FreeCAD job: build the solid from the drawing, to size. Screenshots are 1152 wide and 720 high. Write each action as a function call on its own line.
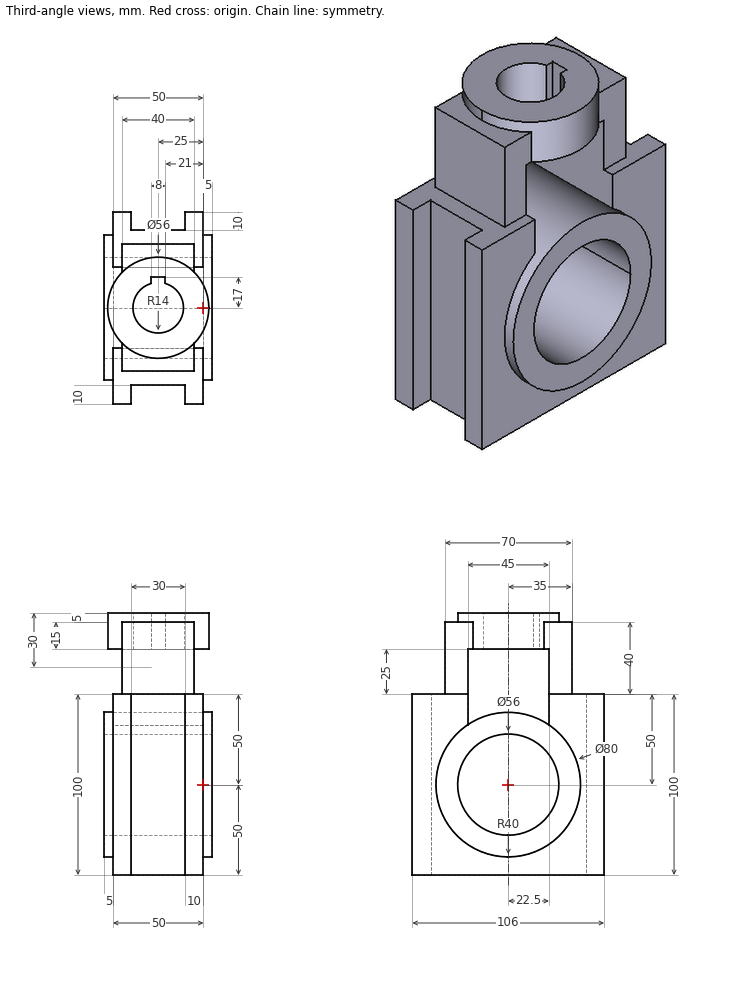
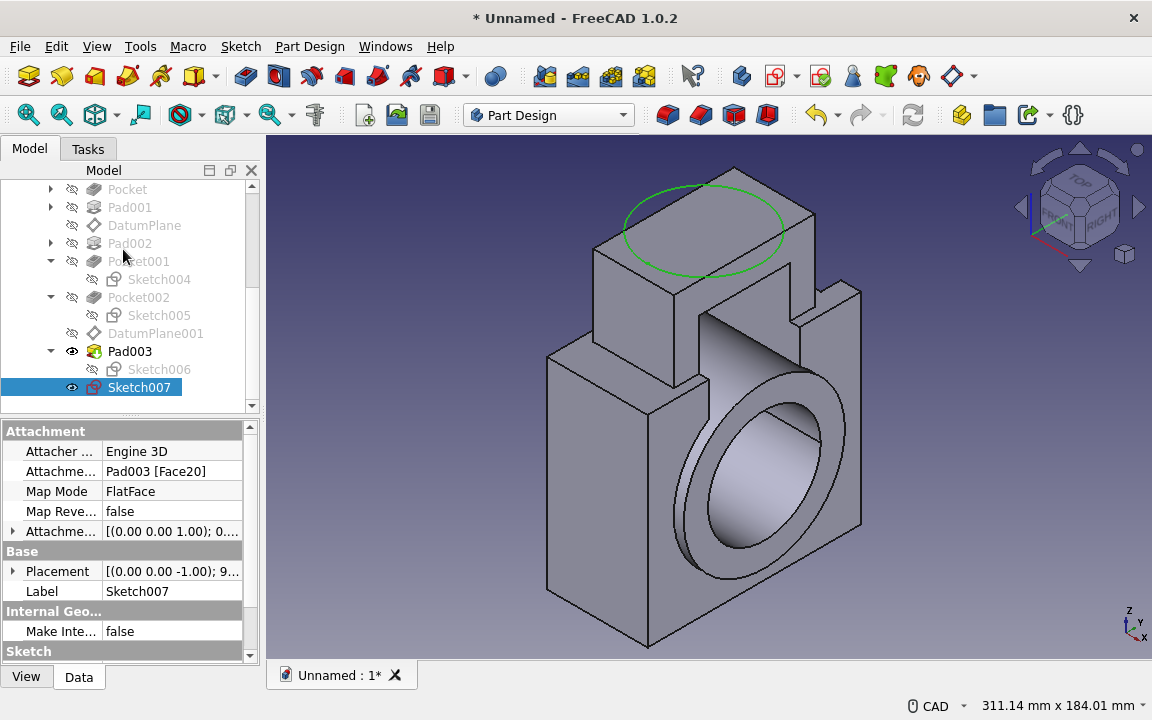
click(246, 76)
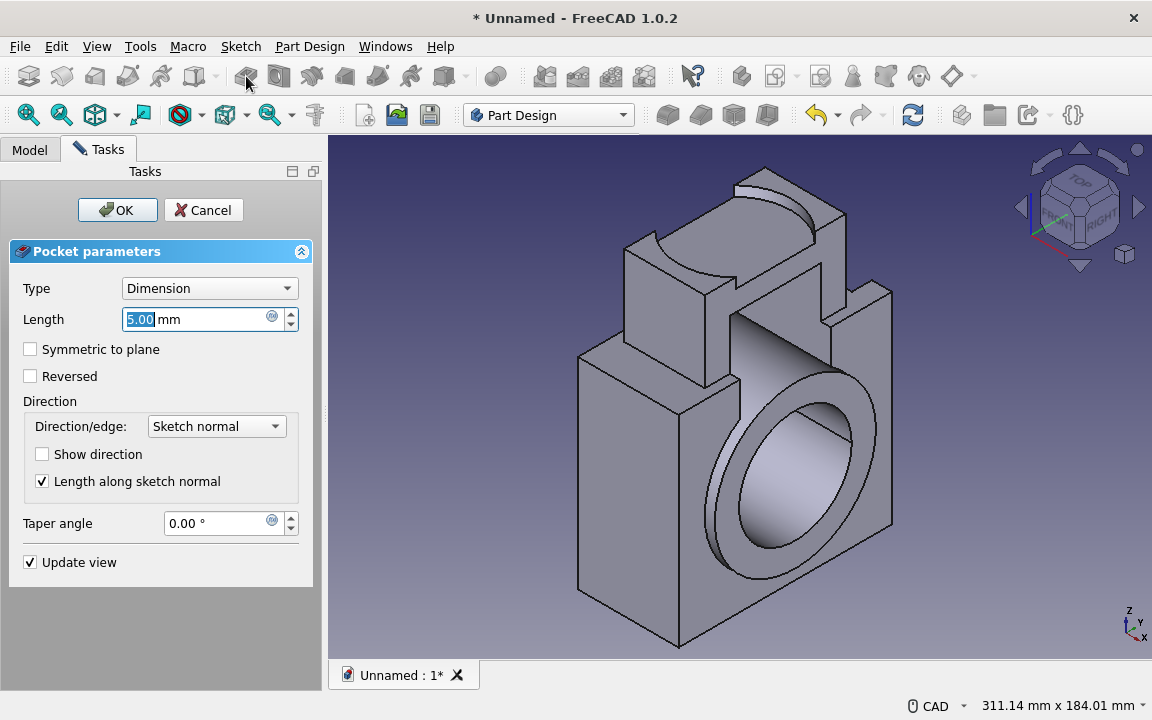
text(15)
key(Tab)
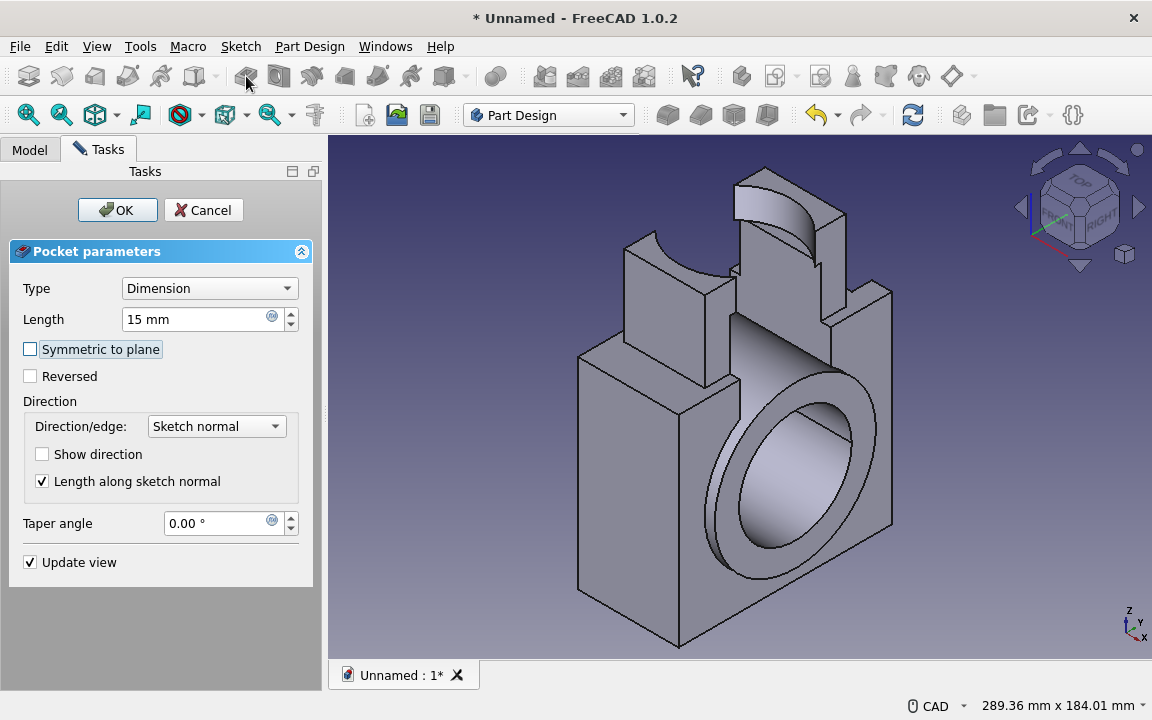
click(118, 210)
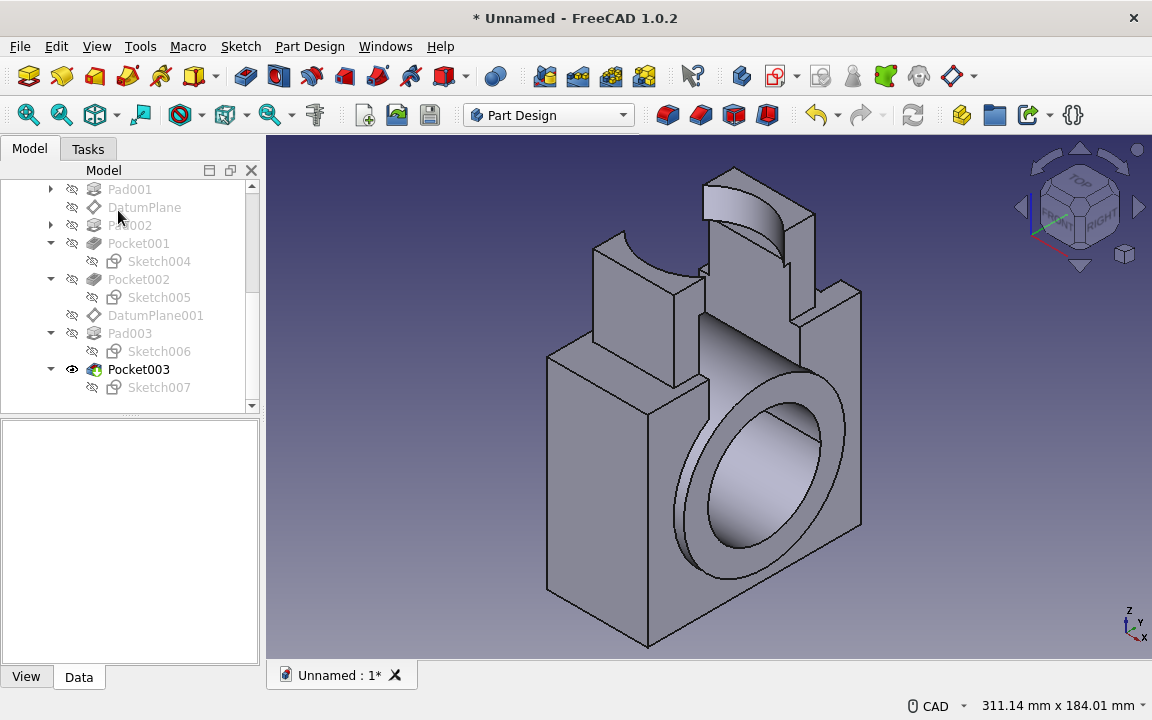
click(622, 251)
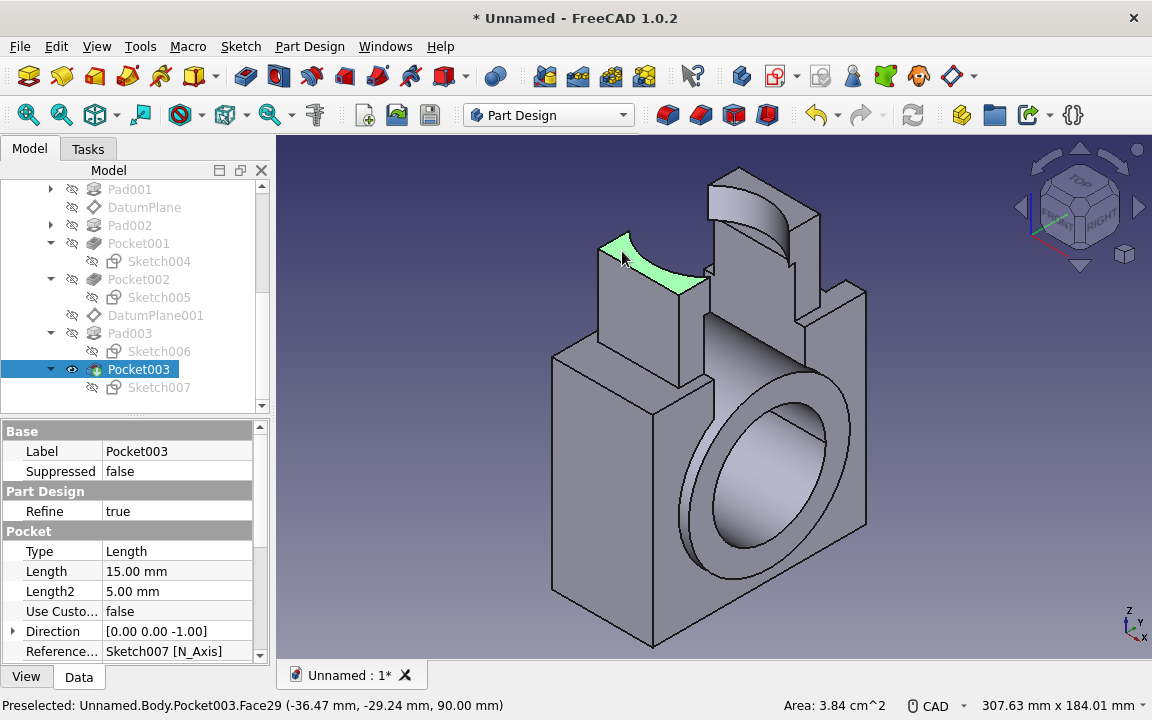
click(774, 76)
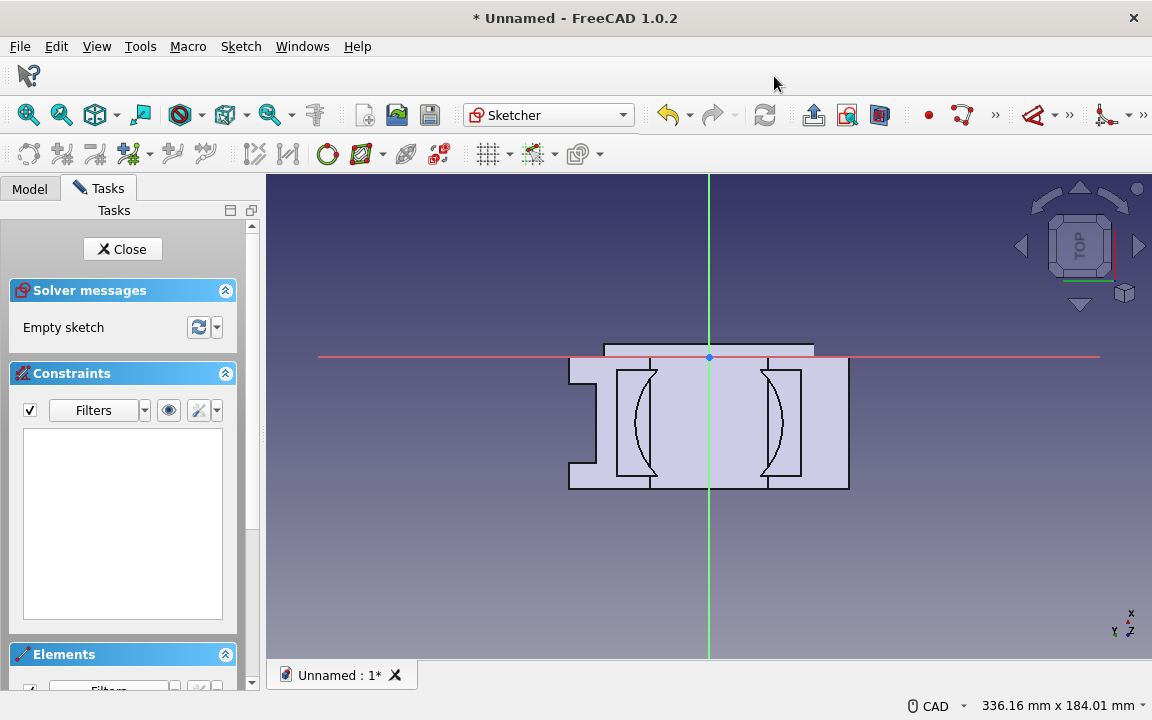
scroll(765, 428, up, 4)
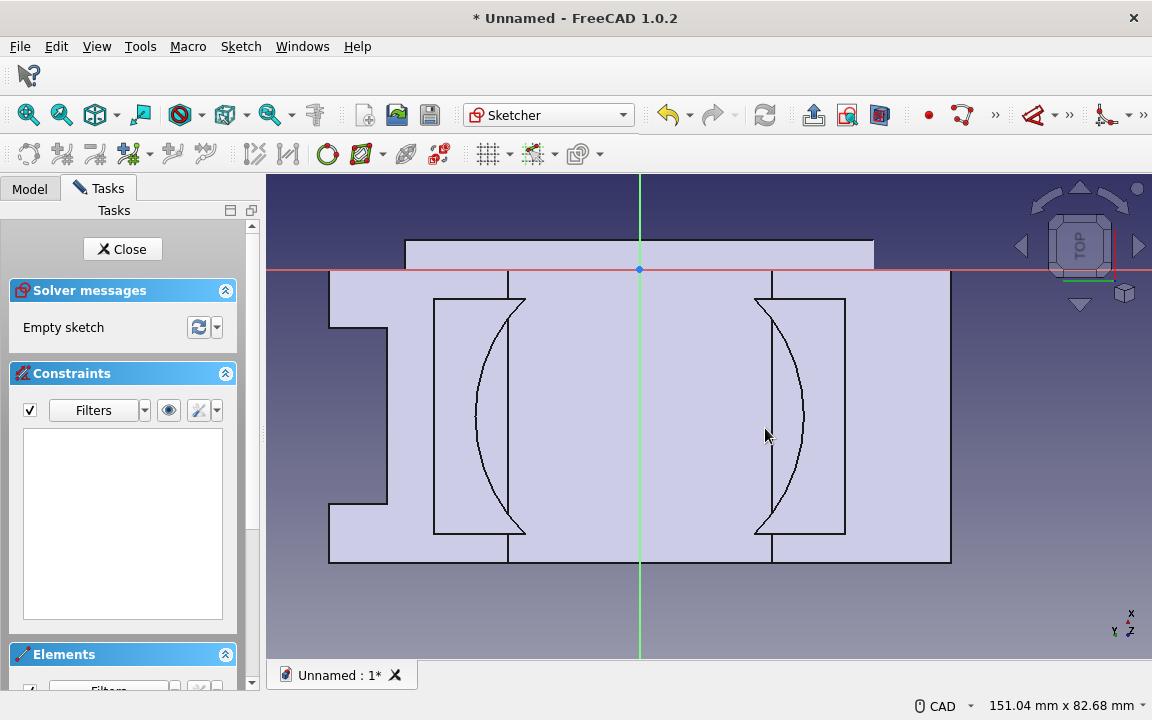
key(g)
key(c)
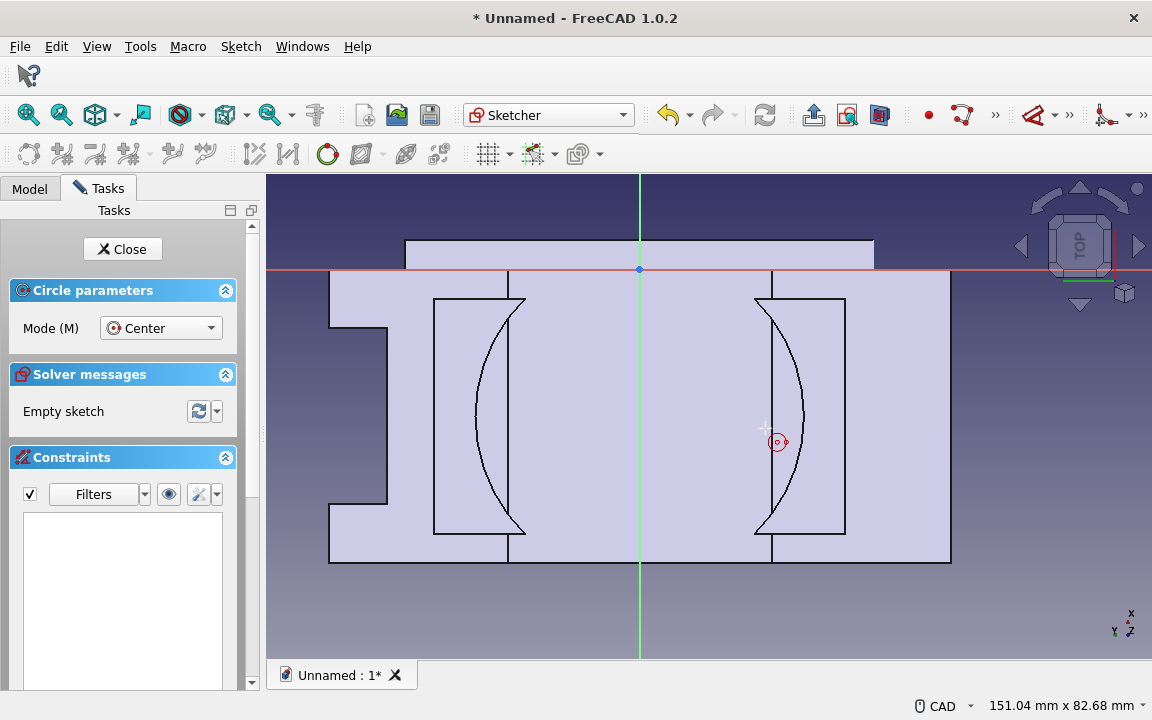
click(640, 416)
move(756, 300)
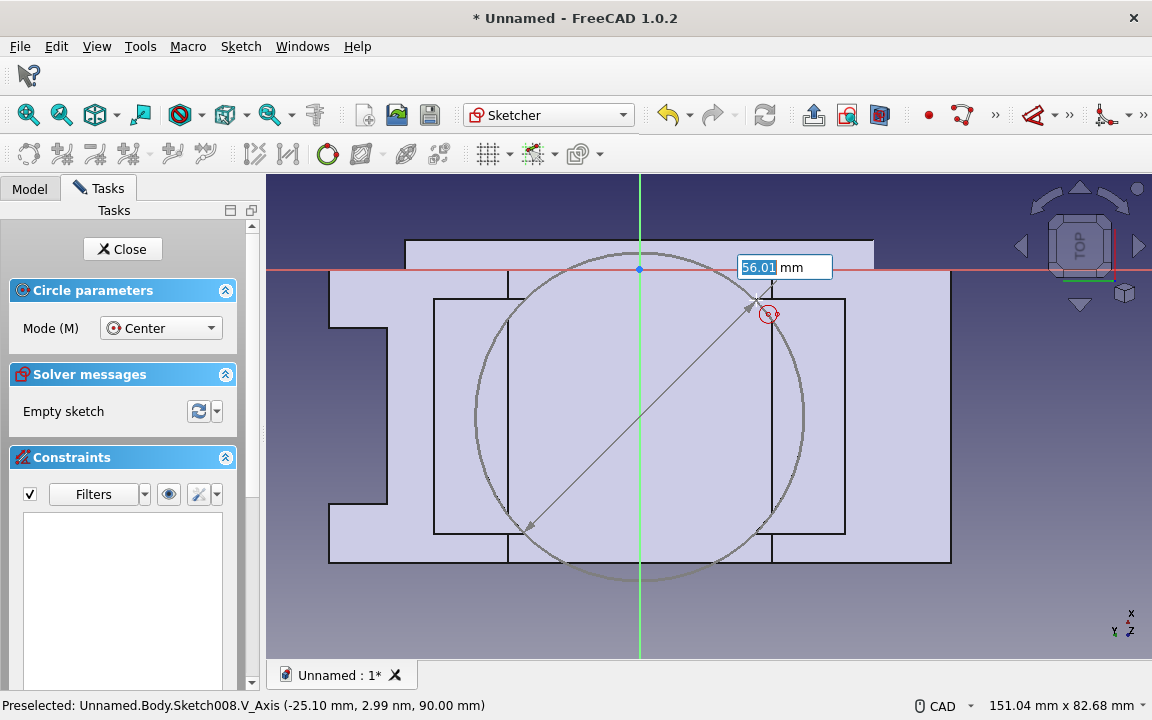
text(56)
key(Return)
key(Escape)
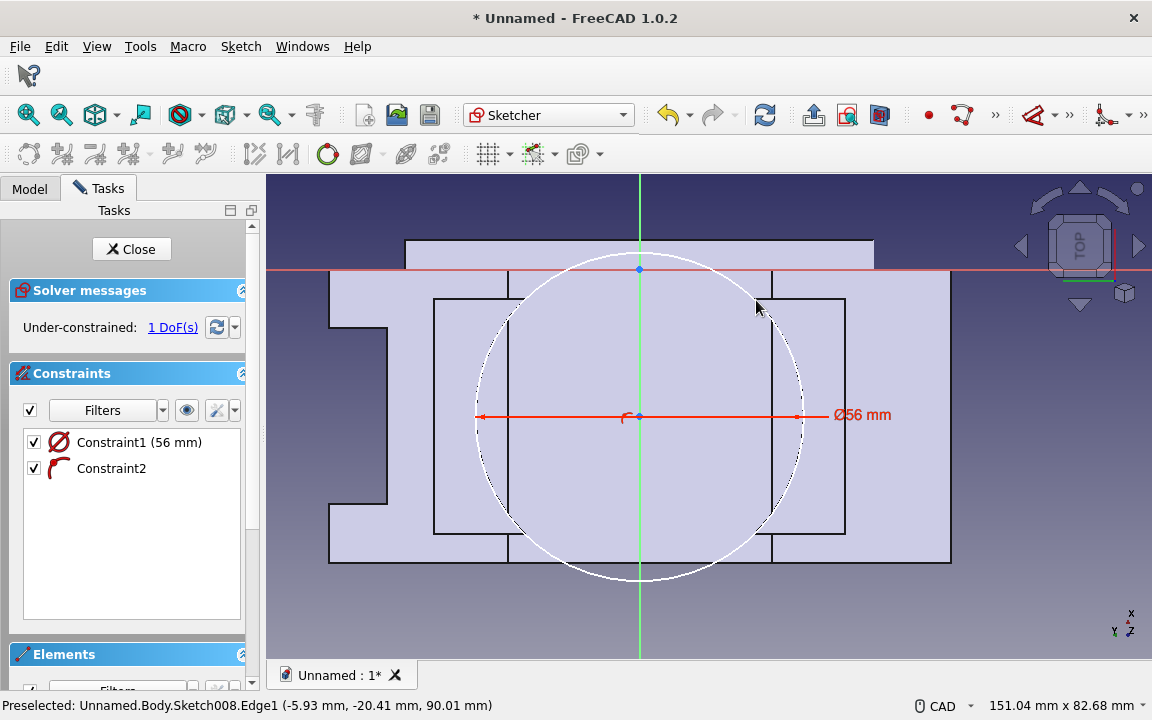
key(d)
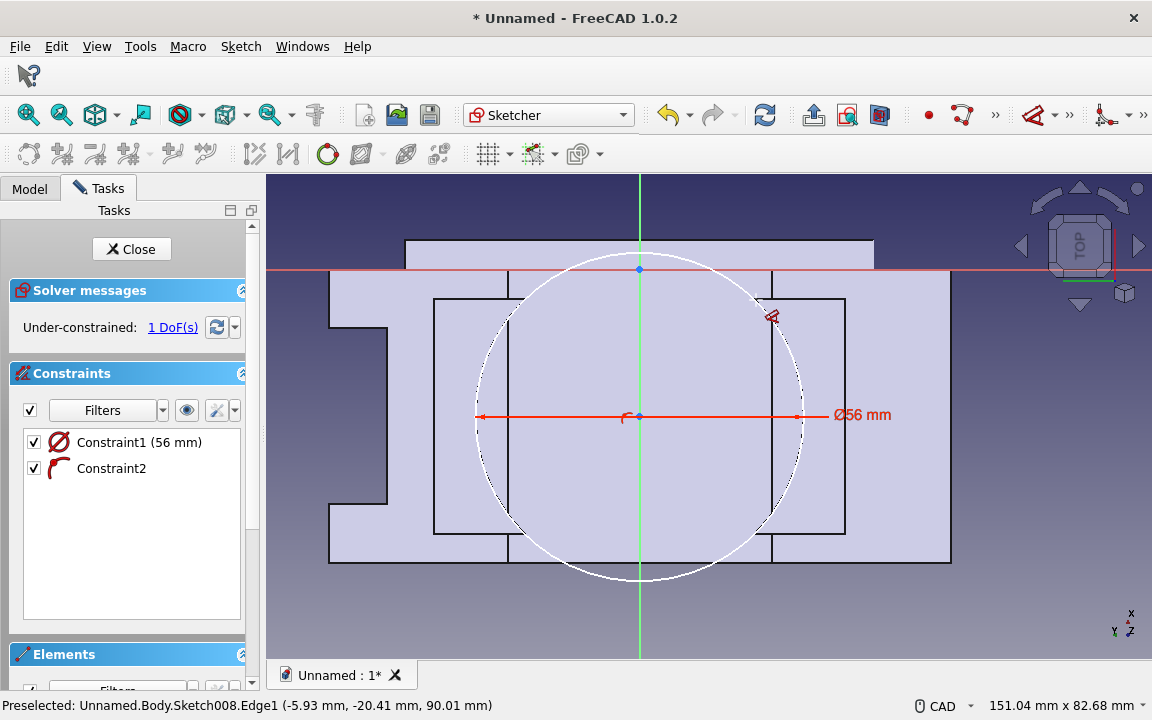
click(640, 417)
click(674, 343)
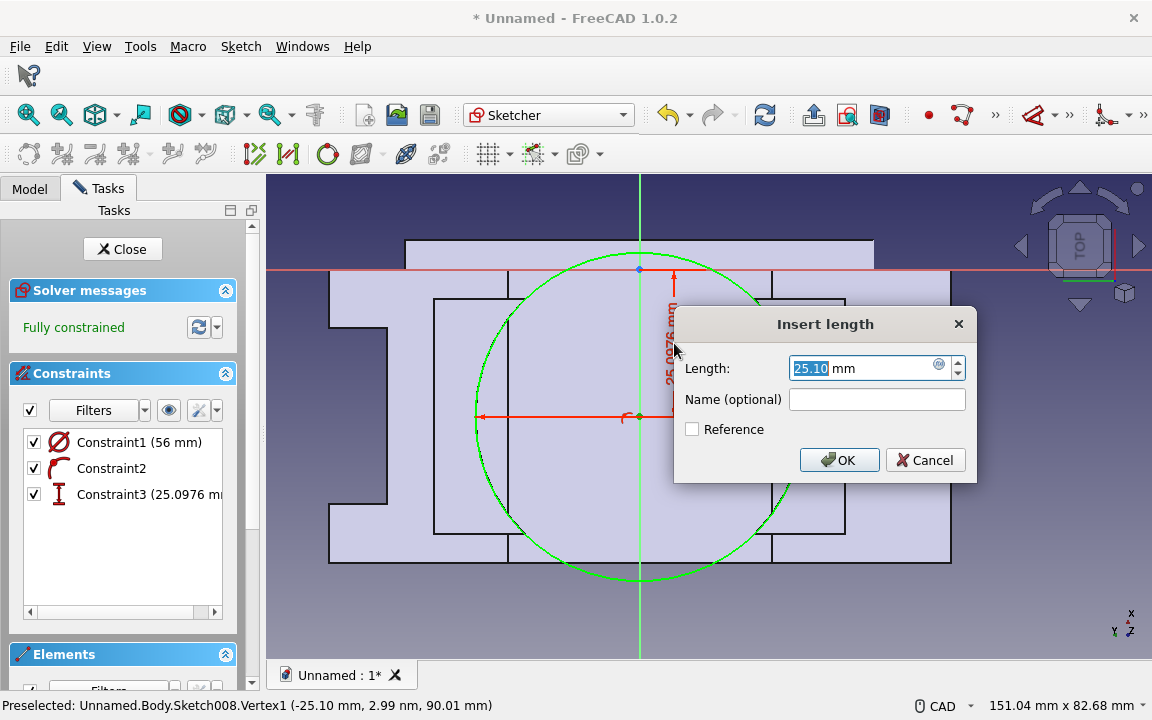
text(25)
key(Return)
key(Escape)